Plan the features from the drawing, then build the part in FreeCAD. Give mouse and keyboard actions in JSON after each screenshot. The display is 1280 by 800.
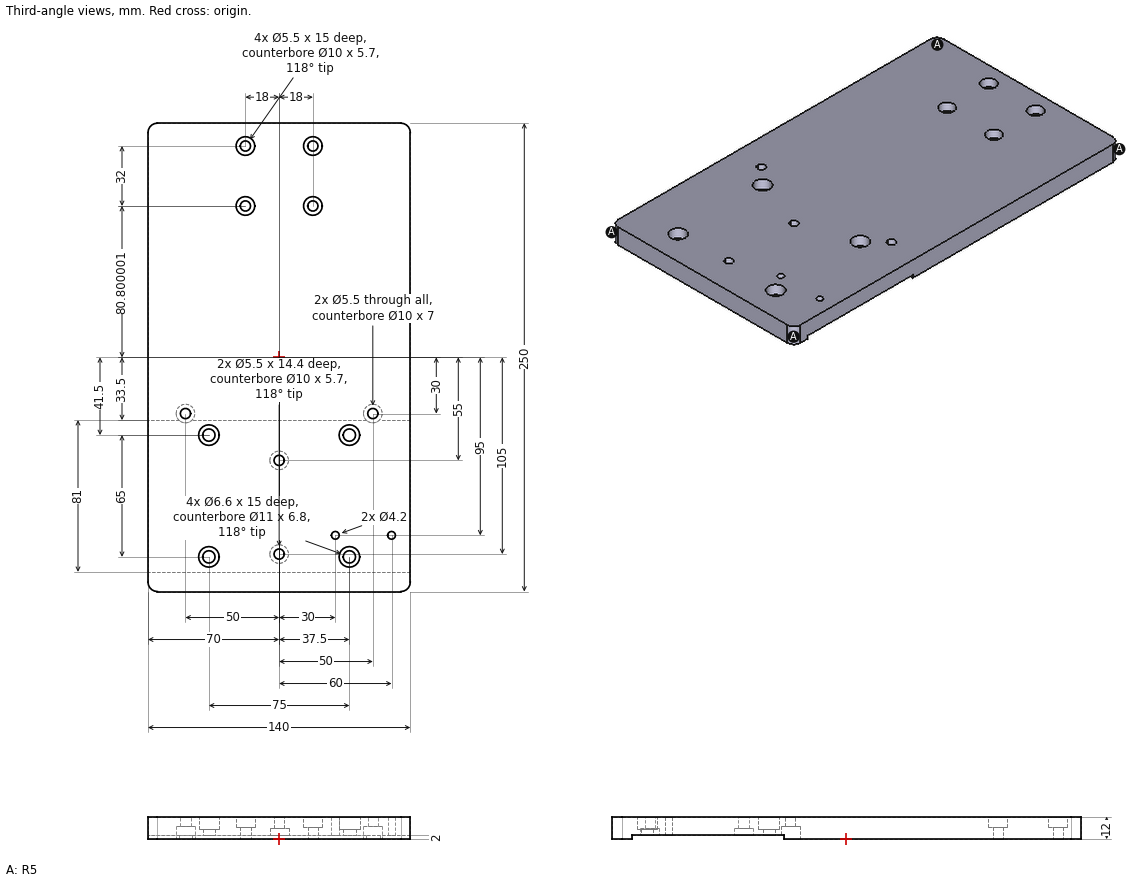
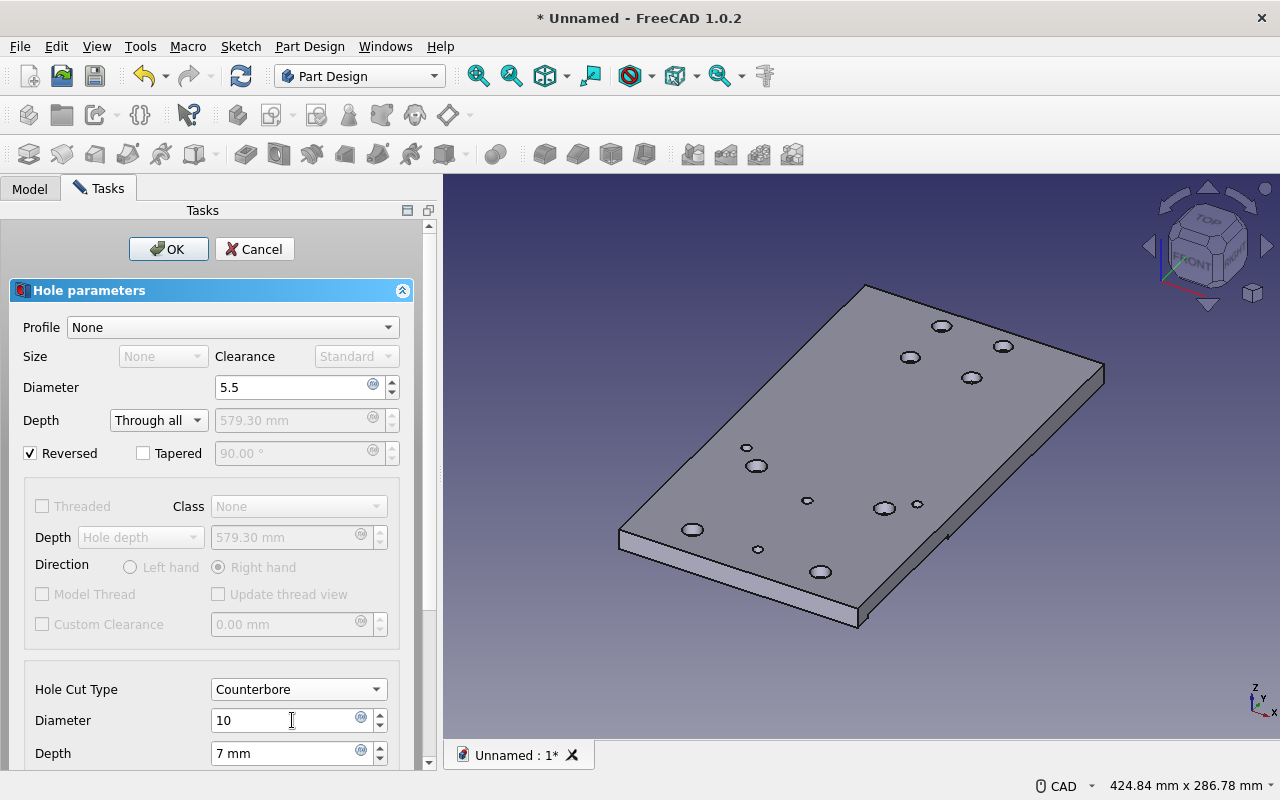
{"action": "left_click", "coordinate": [169, 249]}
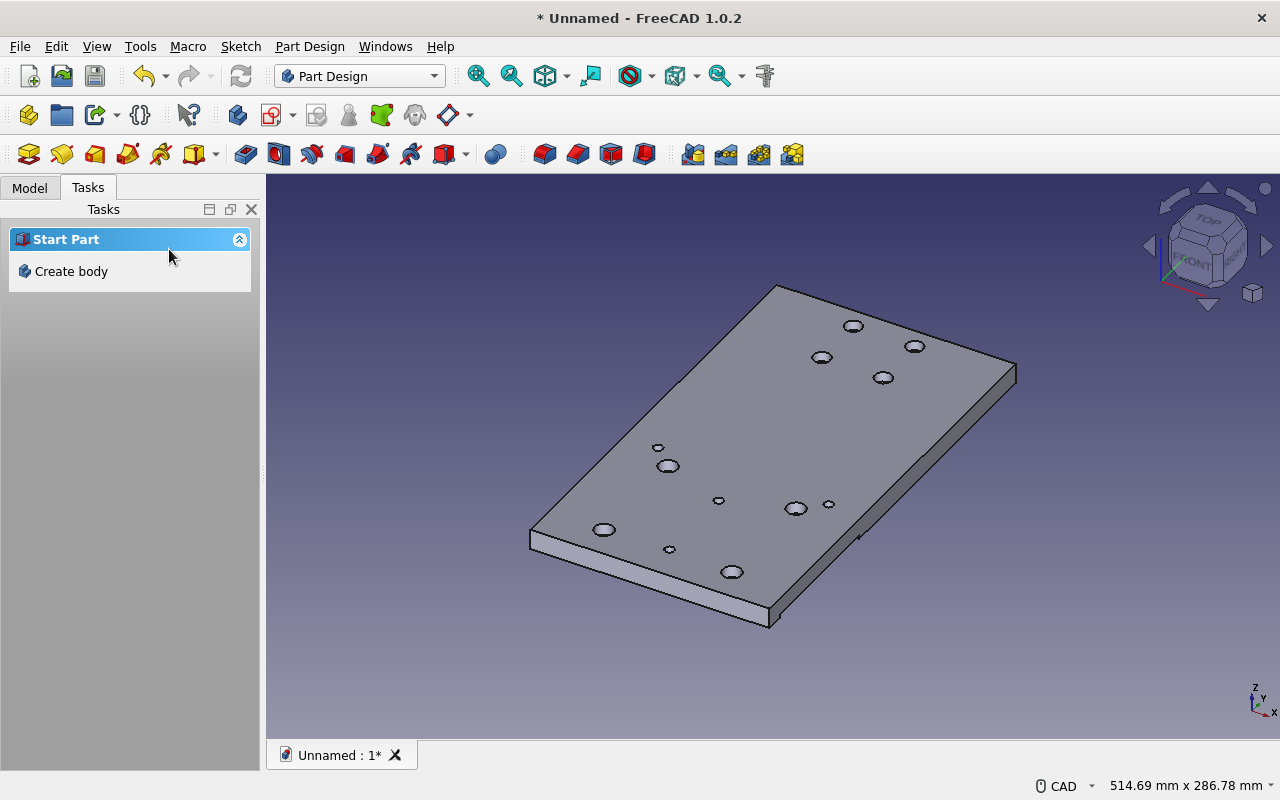
{"action": "left_click", "coordinate": [773, 446]}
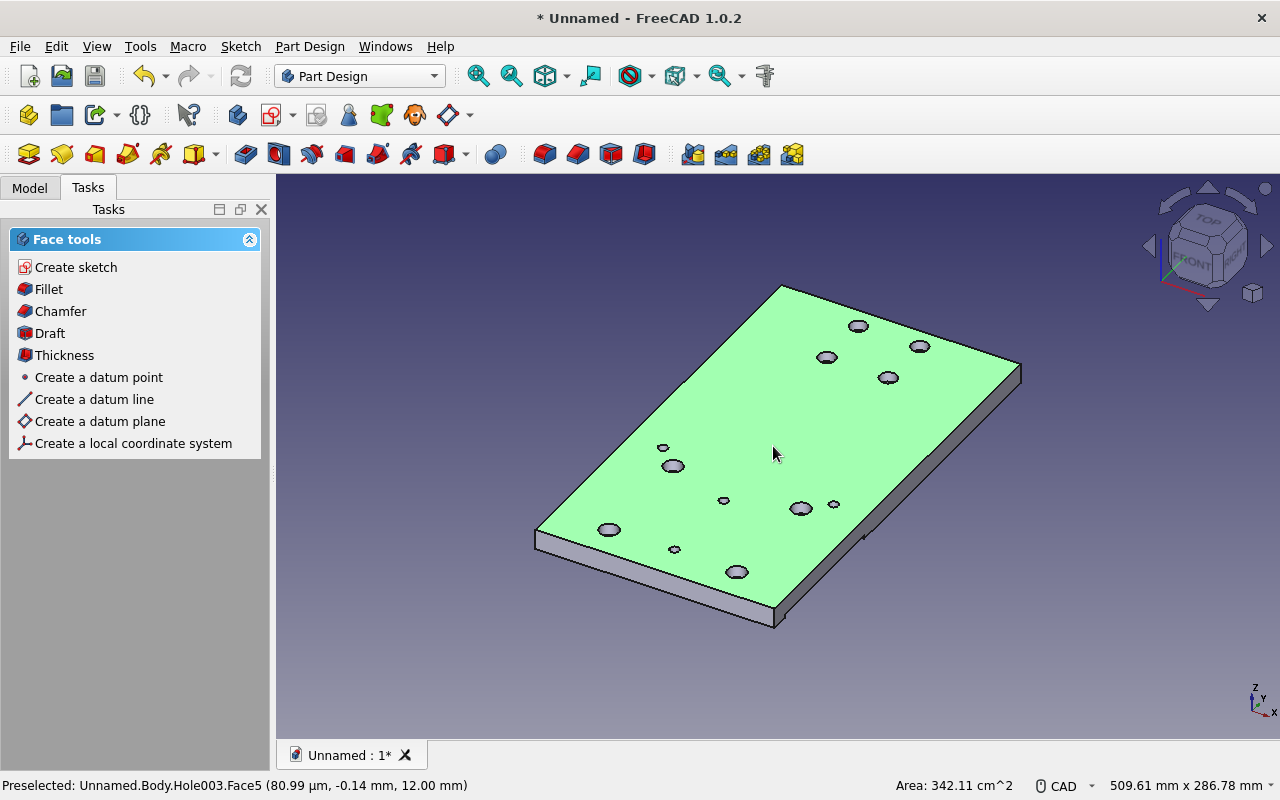
{"action": "left_click", "coordinate": [270, 116]}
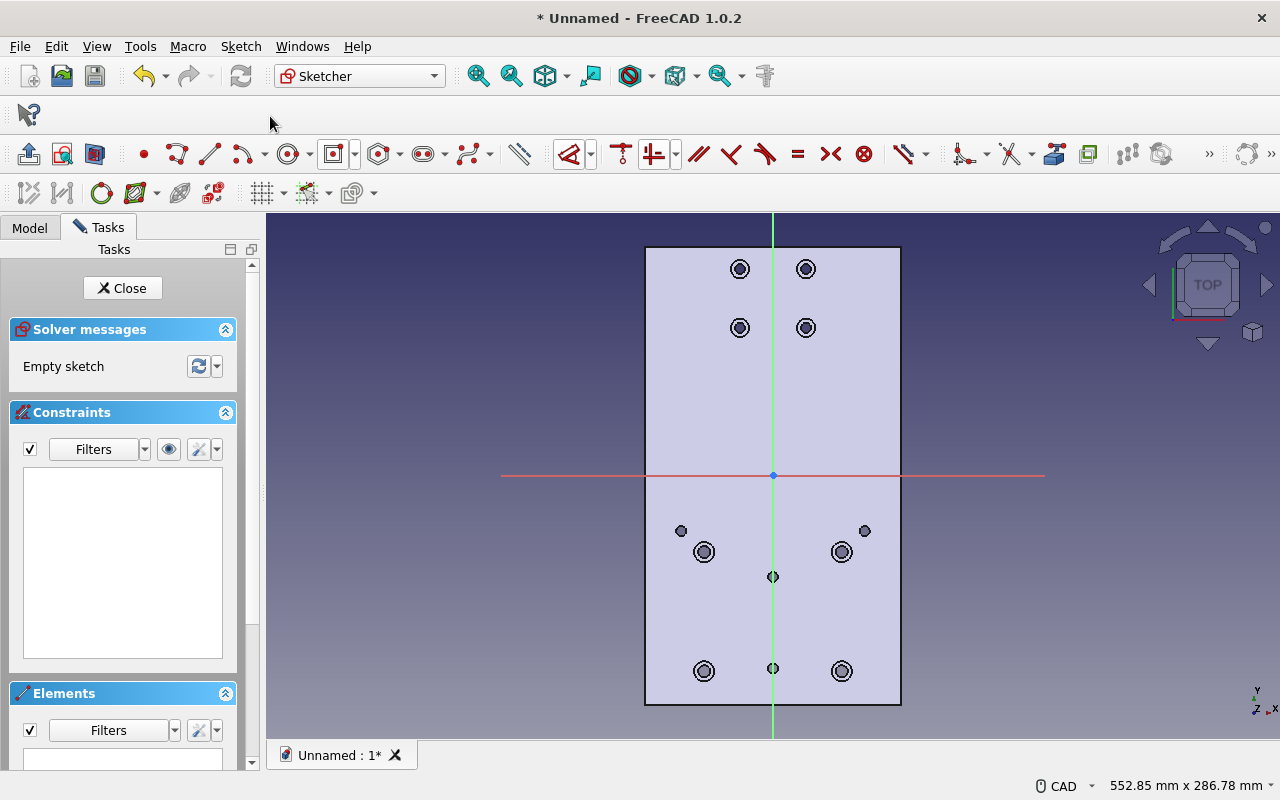
{"action": "scroll", "coordinate": [874, 672], "scroll_direction": "up", "scroll_amount": 11}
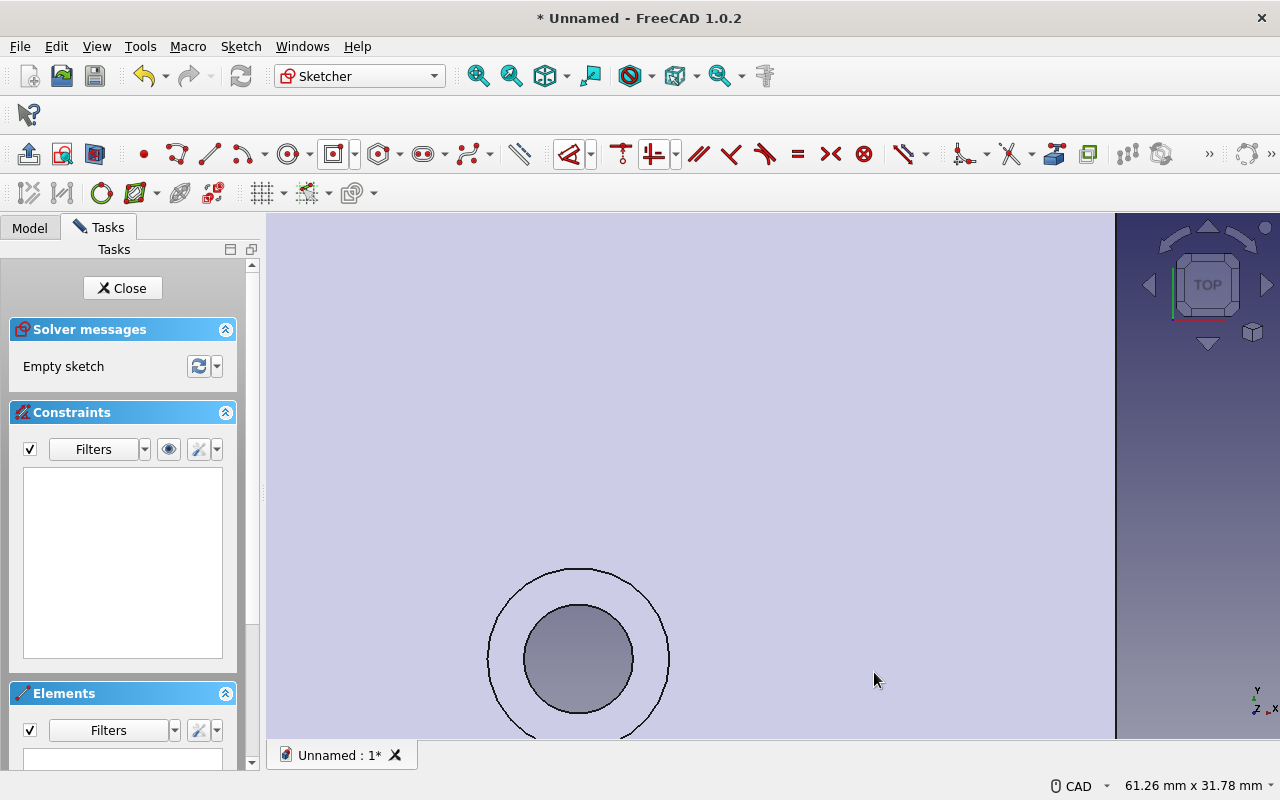
{"action": "left_click", "coordinate": [288, 154]}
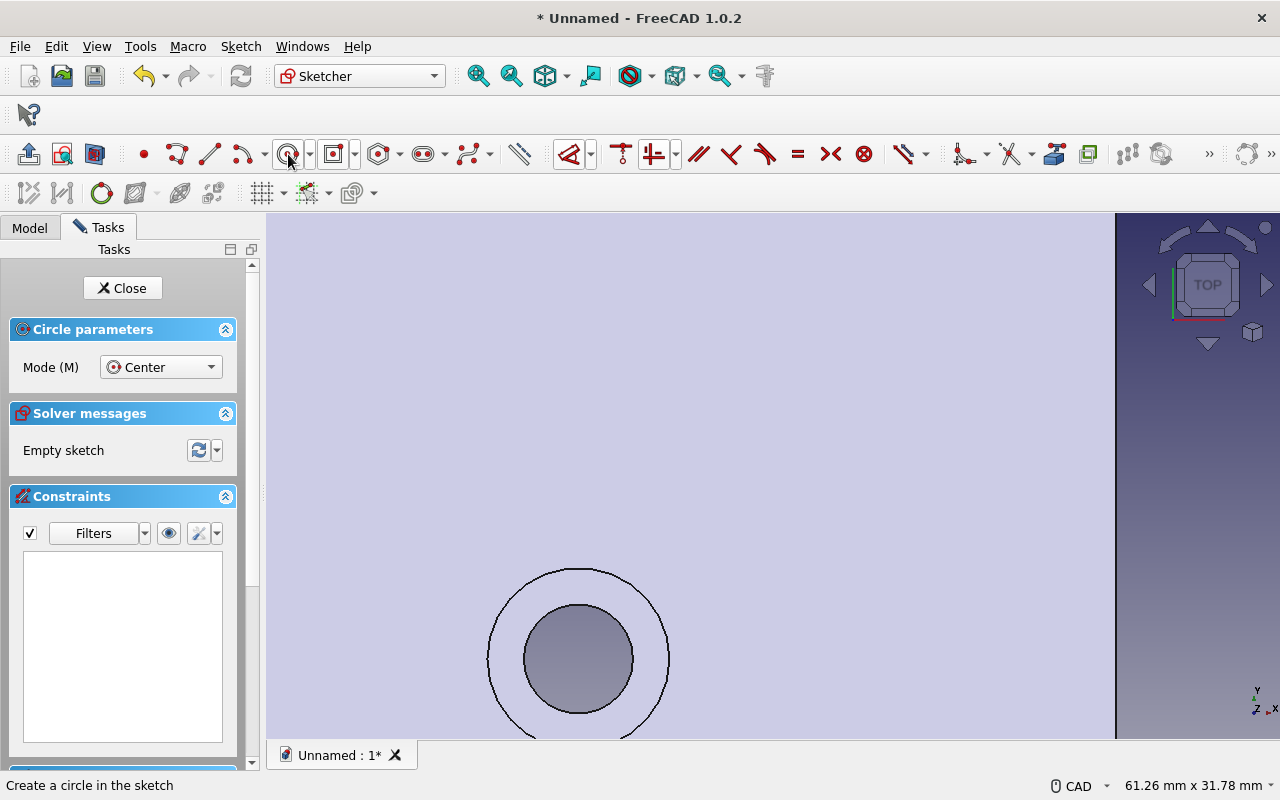
{"action": "left_click", "coordinate": [454, 469]}
{"action": "left_click", "coordinate": [479, 444]}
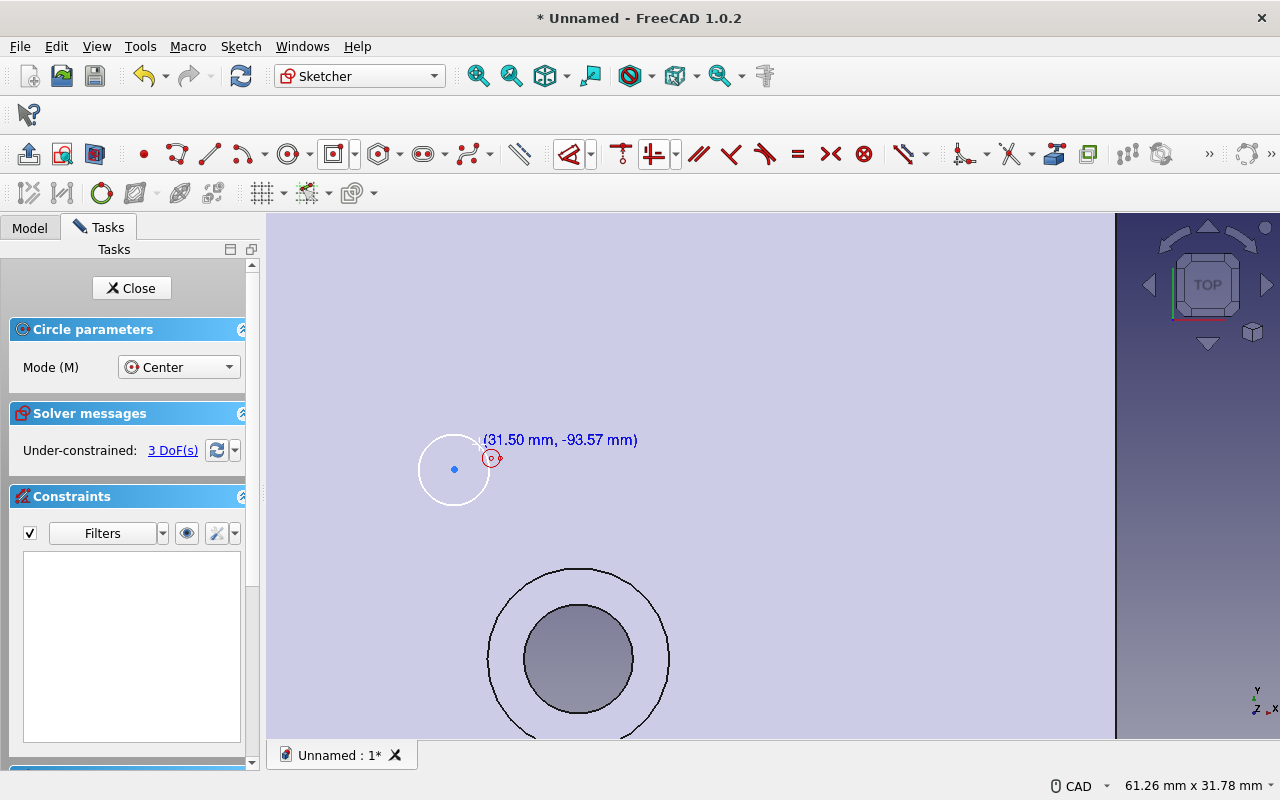
{"action": "left_click", "coordinate": [951, 469]}
{"action": "left_click", "coordinate": [975, 444]}
{"action": "key", "text": "Escape"}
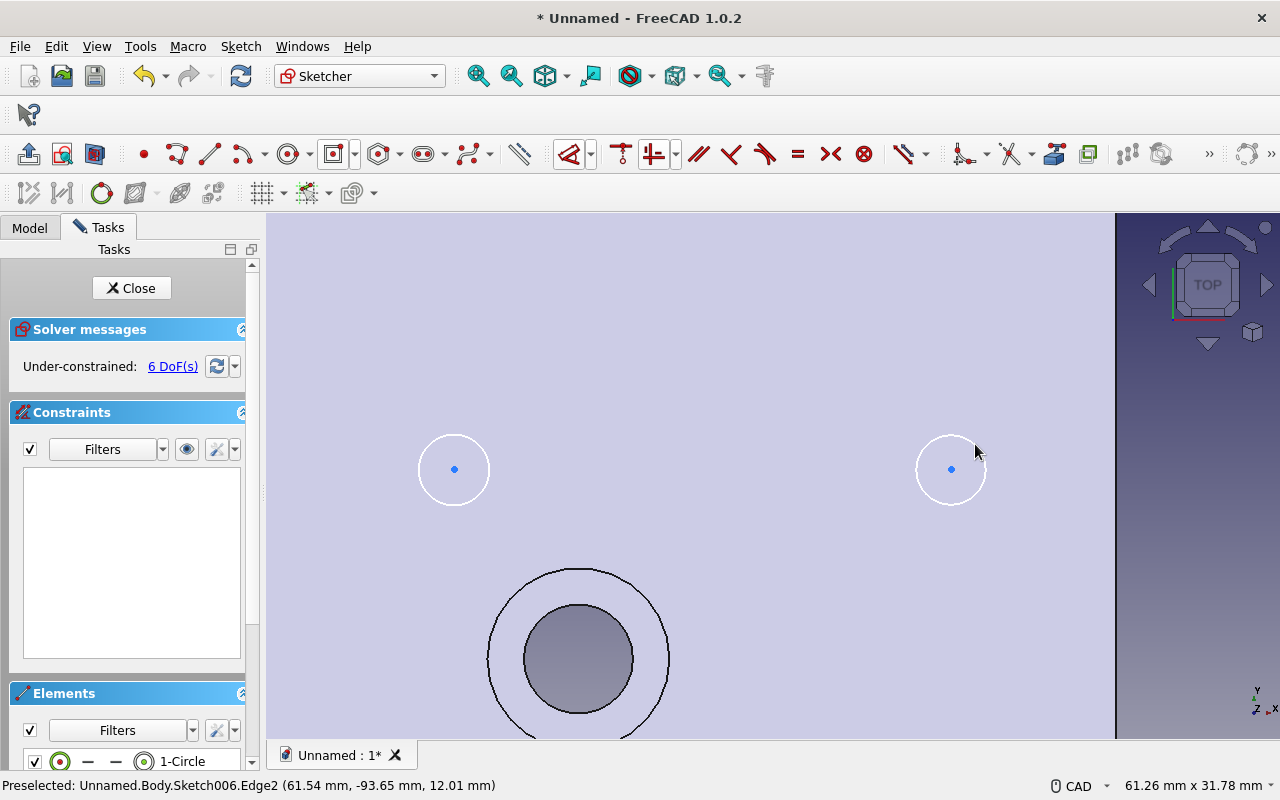
{"action": "left_click", "coordinate": [479, 445]}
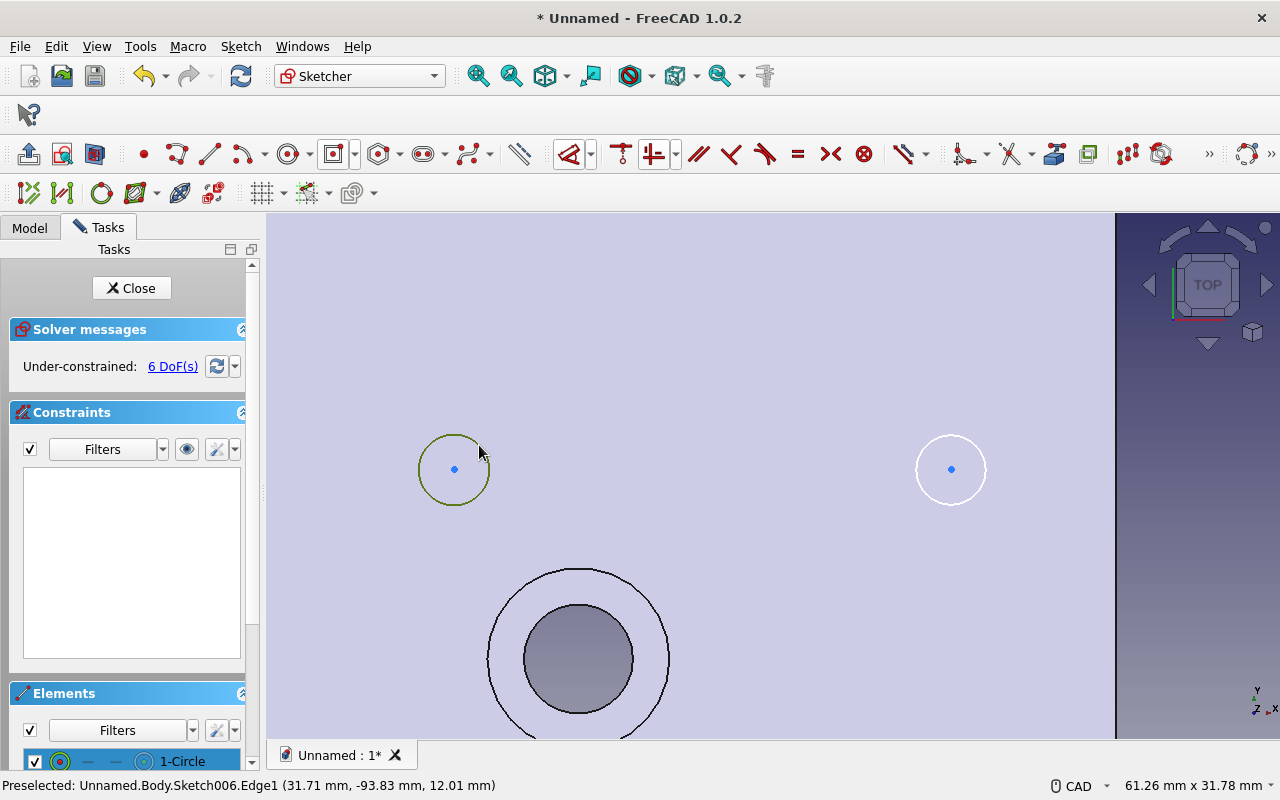
{"action": "left_click", "coordinate": [975, 445]}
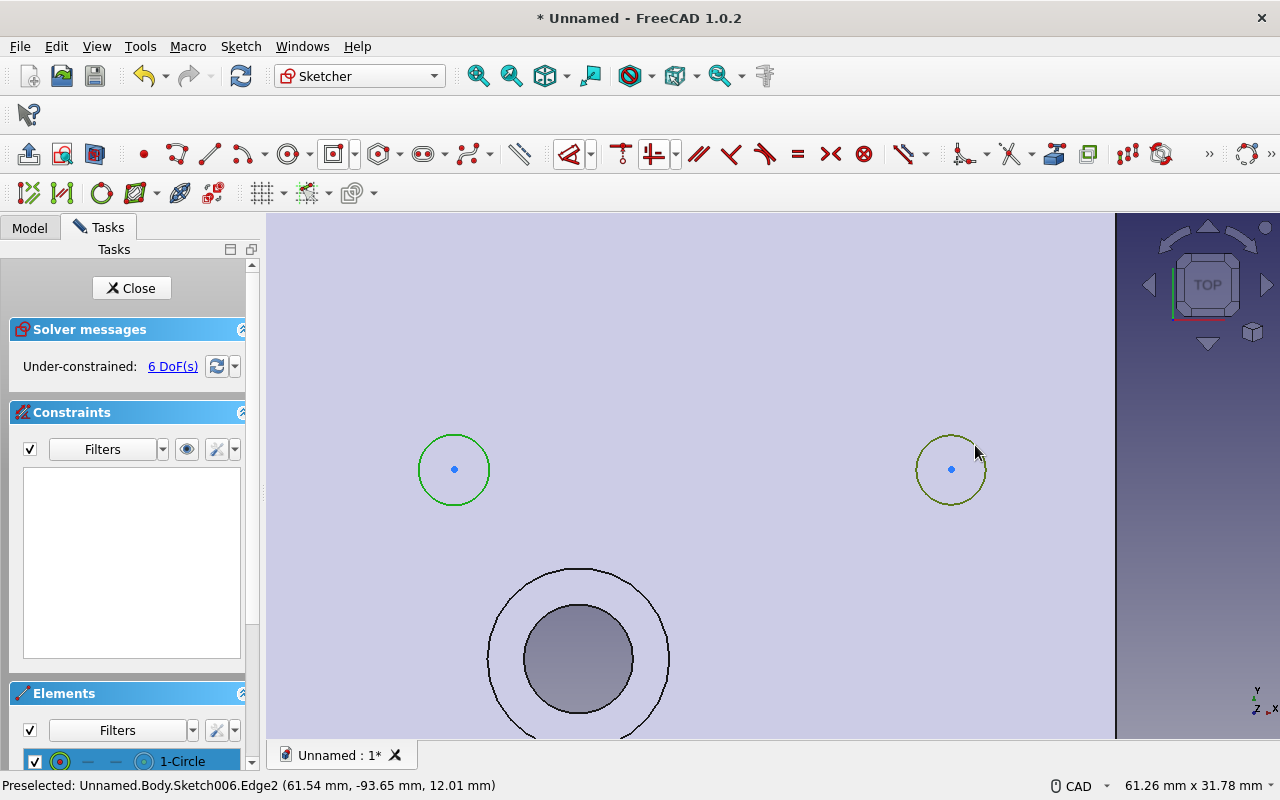
{"action": "key", "text": "e"}